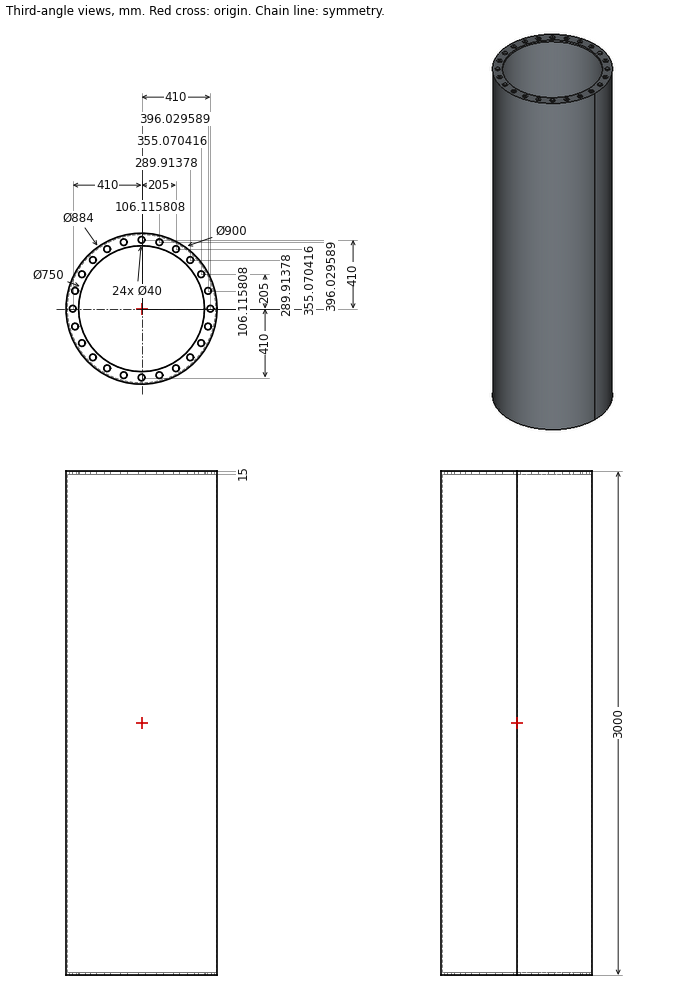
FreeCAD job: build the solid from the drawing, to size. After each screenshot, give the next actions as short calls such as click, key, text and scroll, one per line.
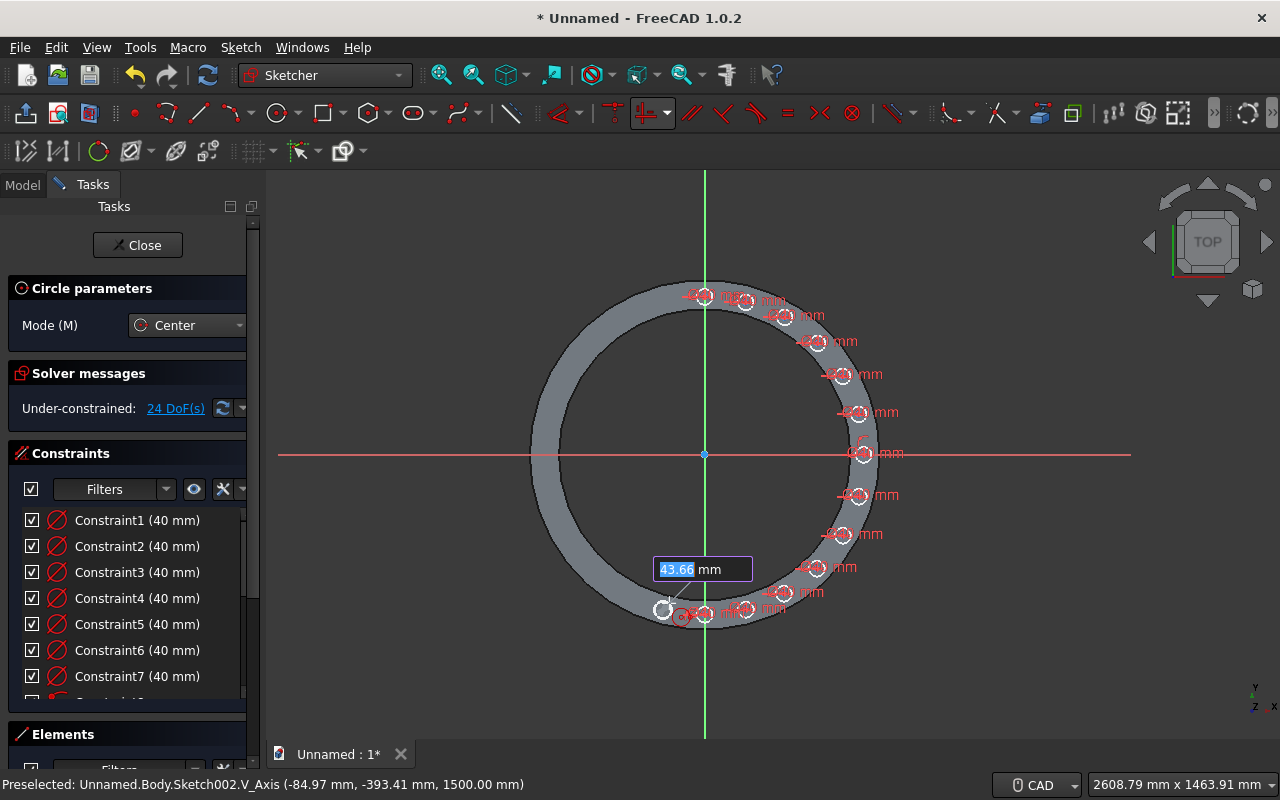
text(40)
key(Return)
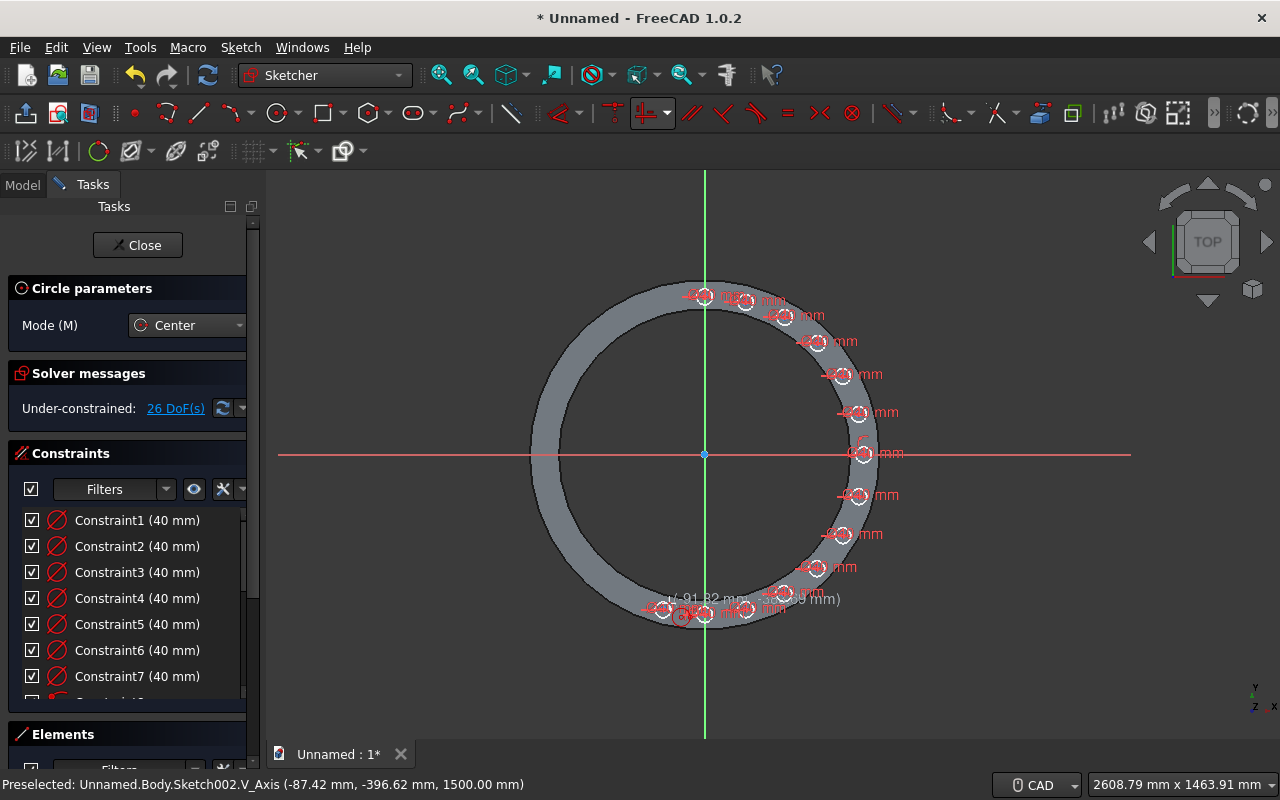
scroll(625, 593, up, 6)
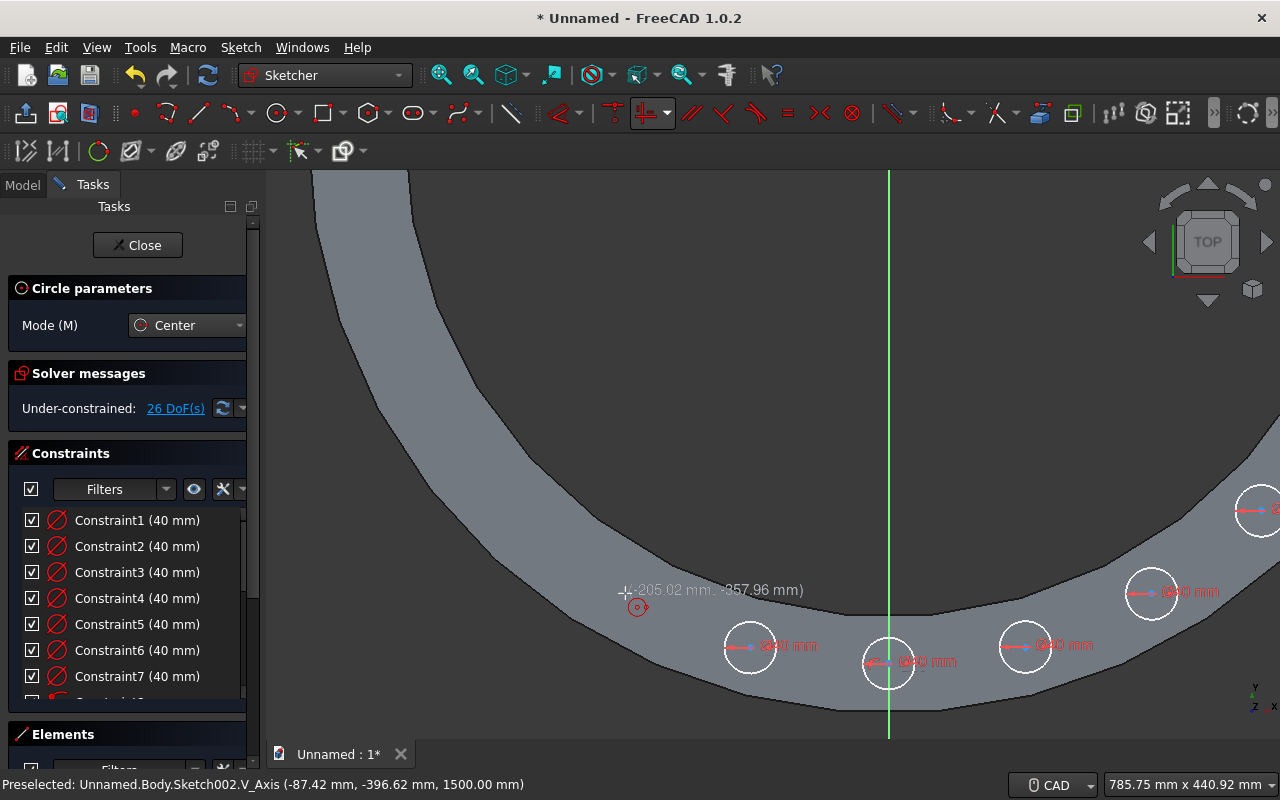
scroll(625, 593, down, 6)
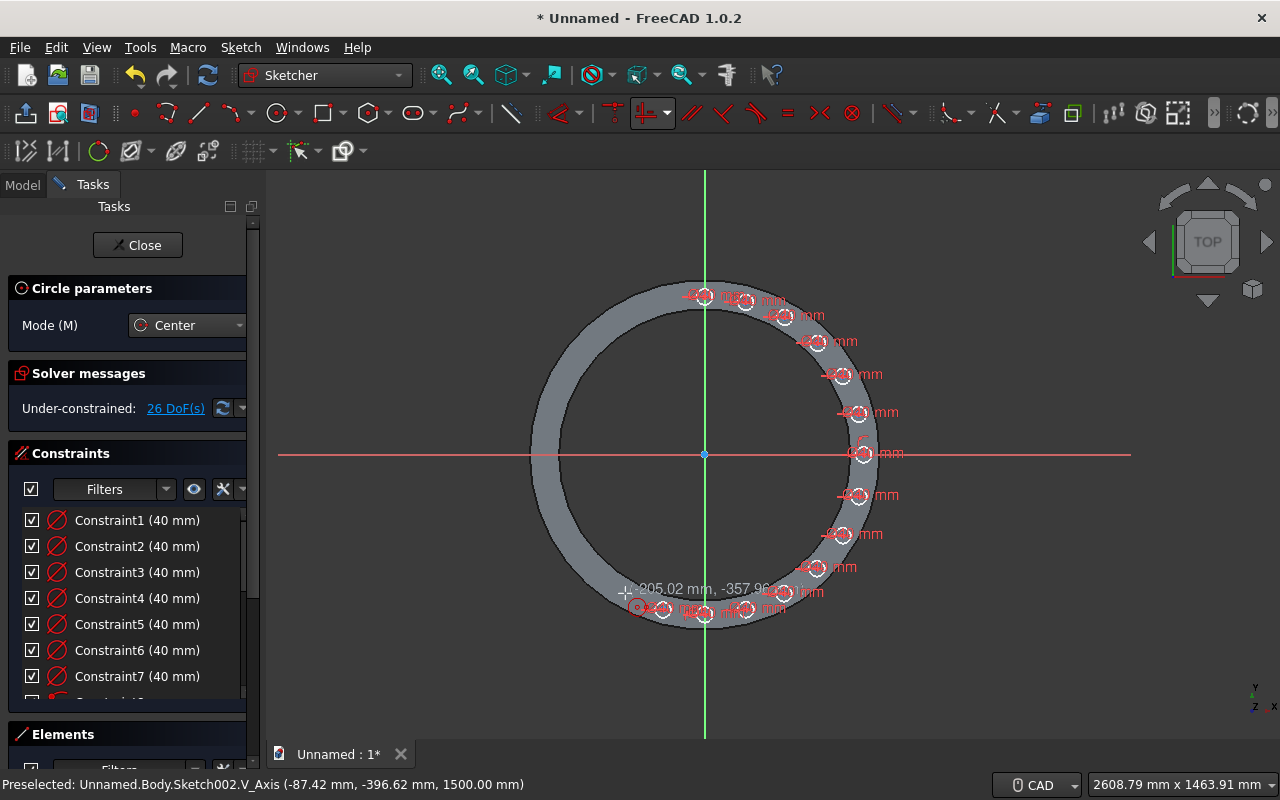
click(625, 593)
move(631, 587)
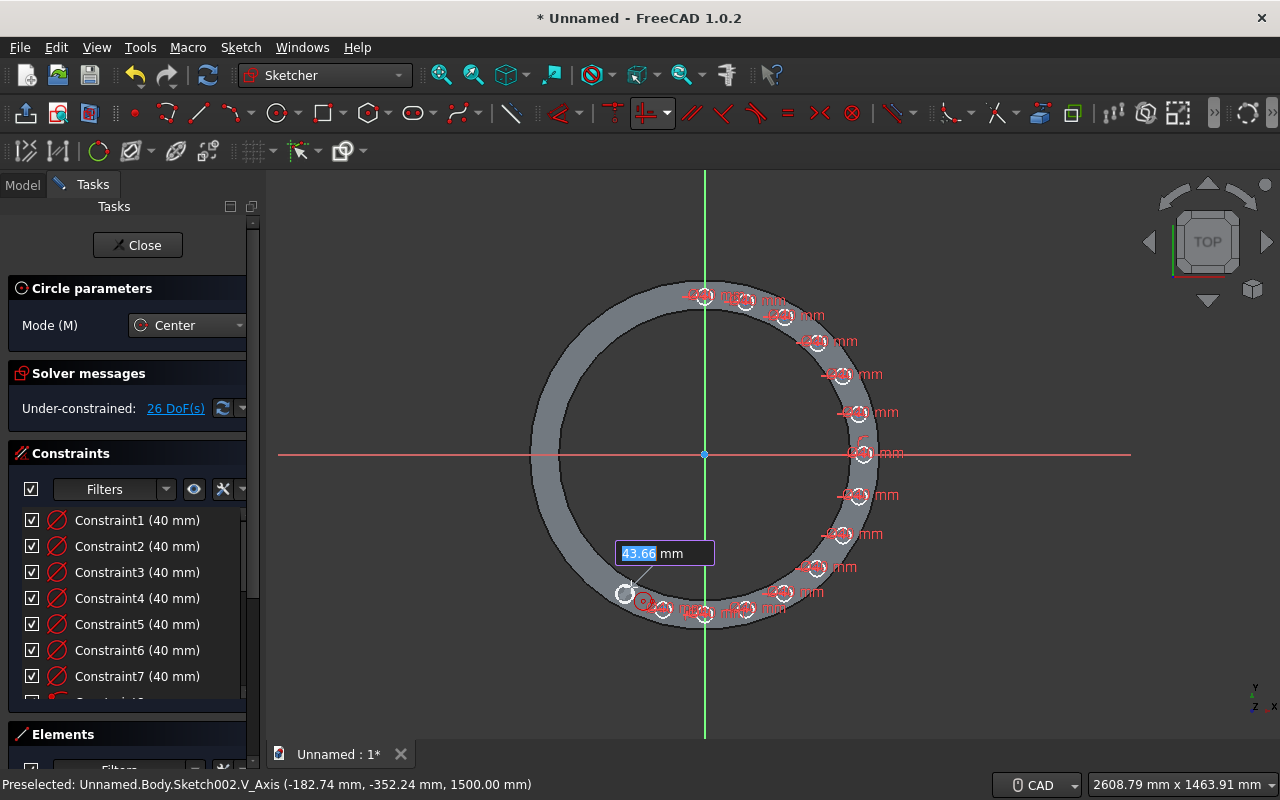
text(40)
key(Return)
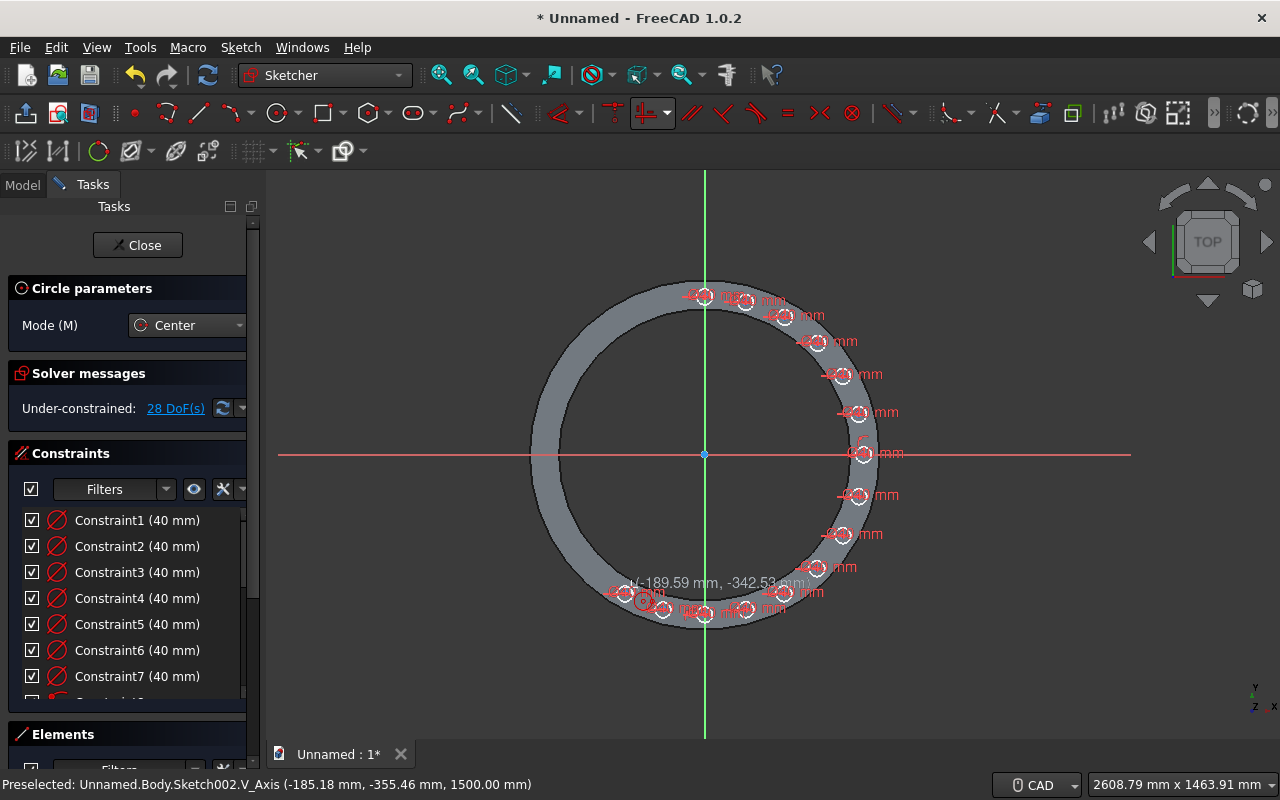
scroll(592, 568, up, 6)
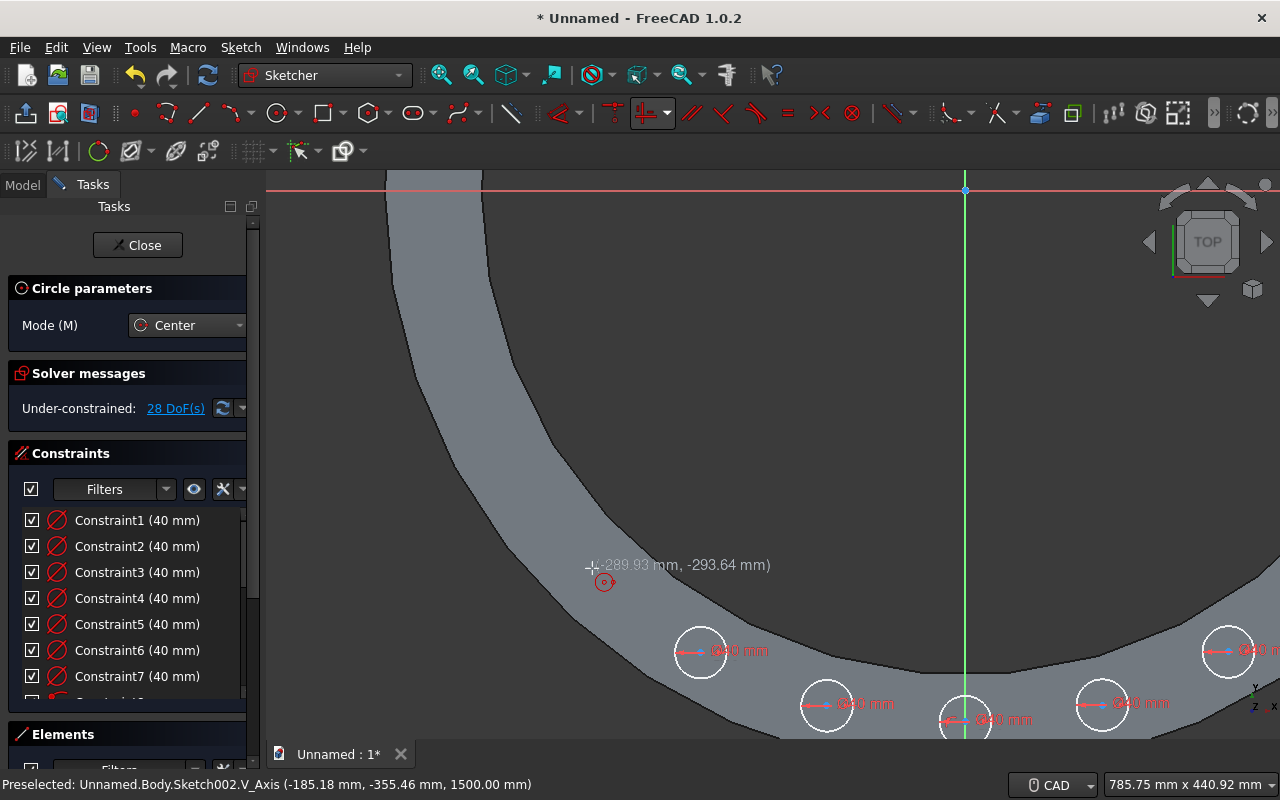
scroll(592, 568, down, 6)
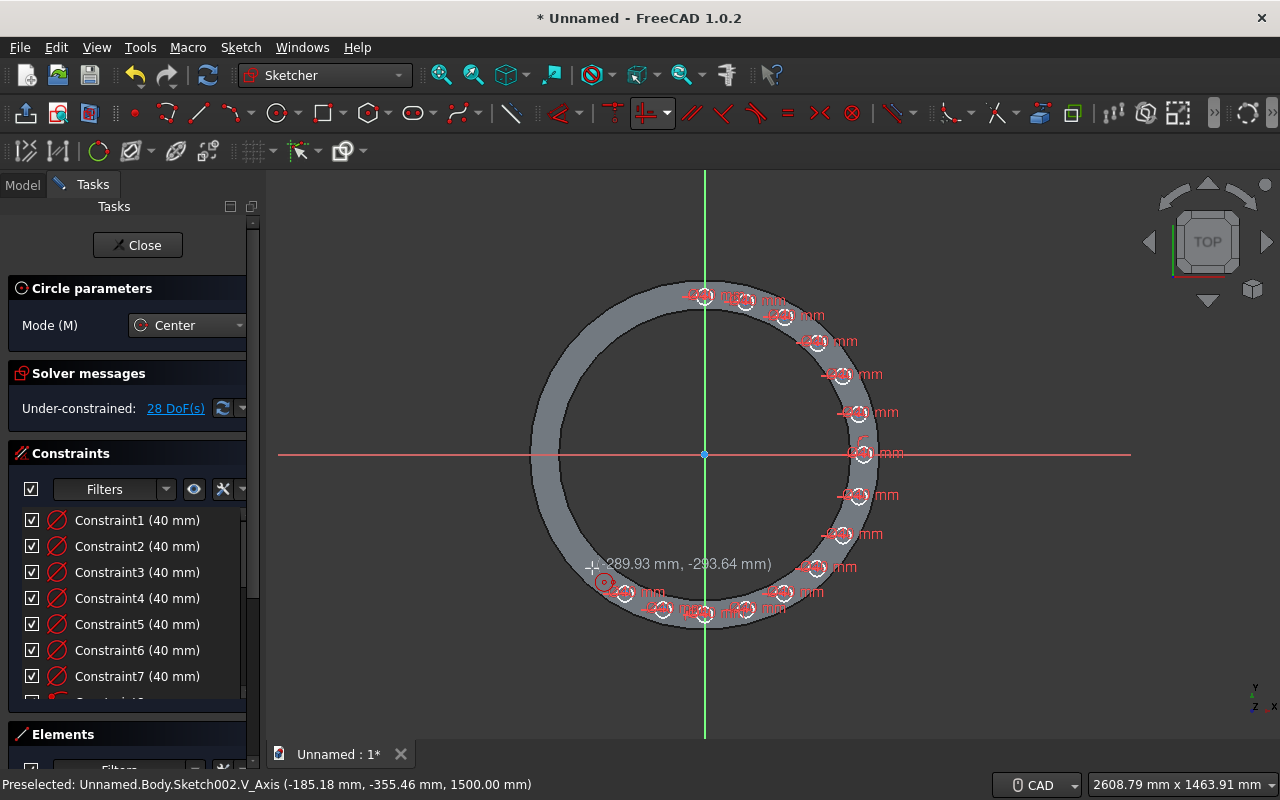
click(592, 568)
move(598, 562)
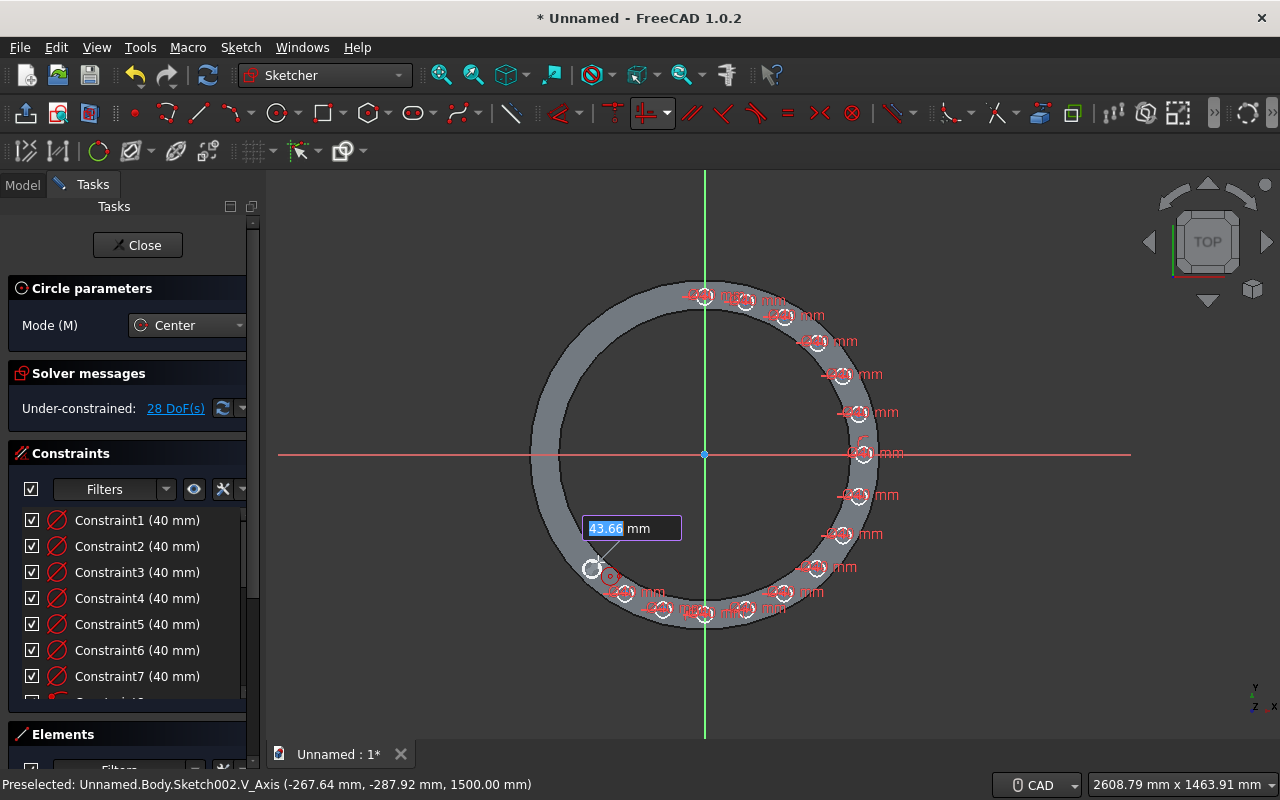
text(40)
key(Return)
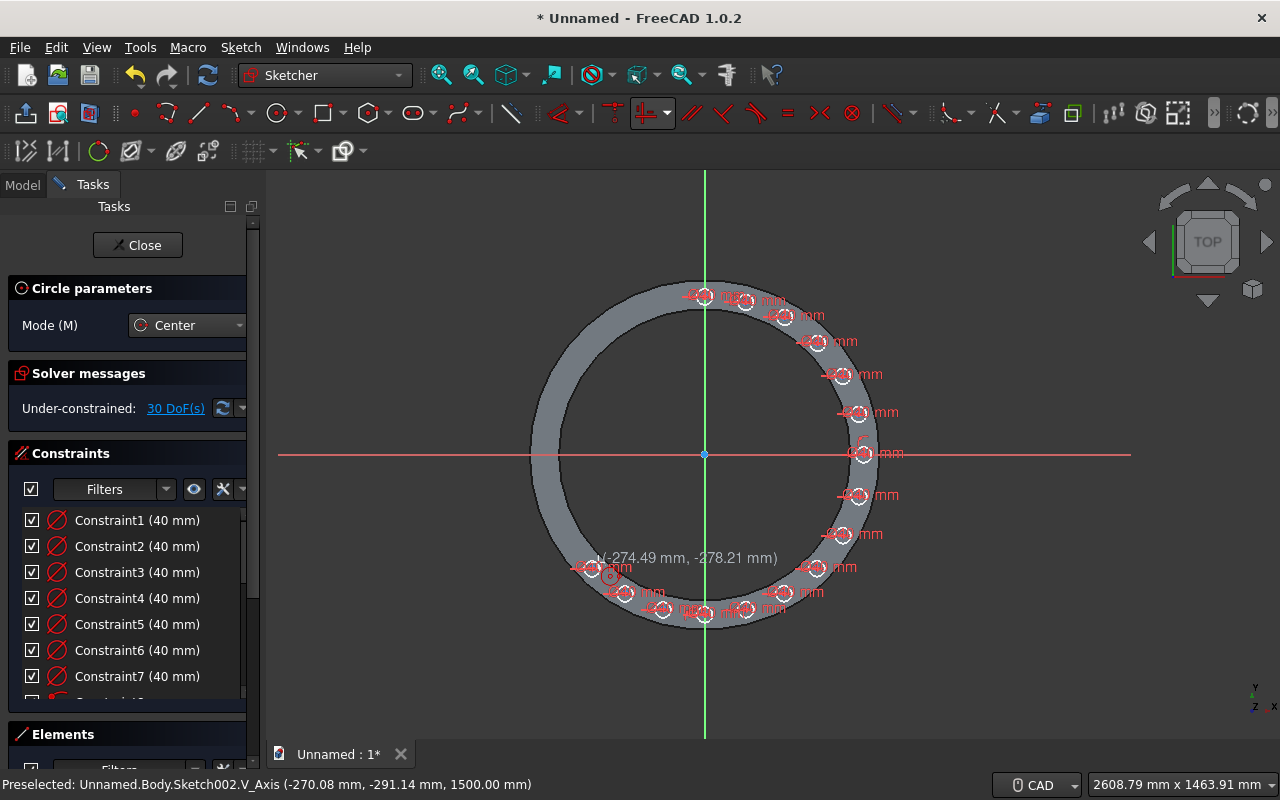
scroll(567, 535, up, 6)